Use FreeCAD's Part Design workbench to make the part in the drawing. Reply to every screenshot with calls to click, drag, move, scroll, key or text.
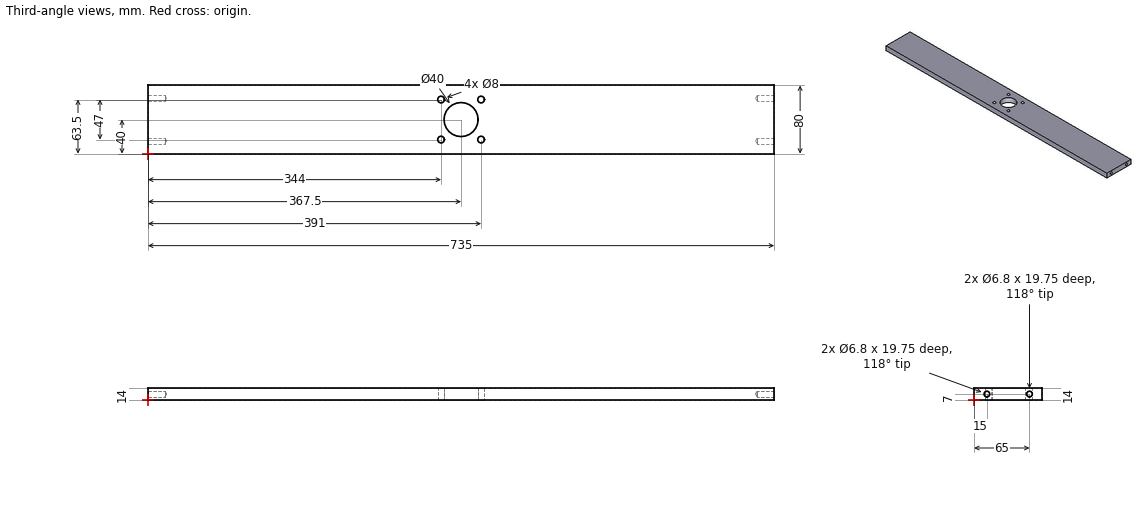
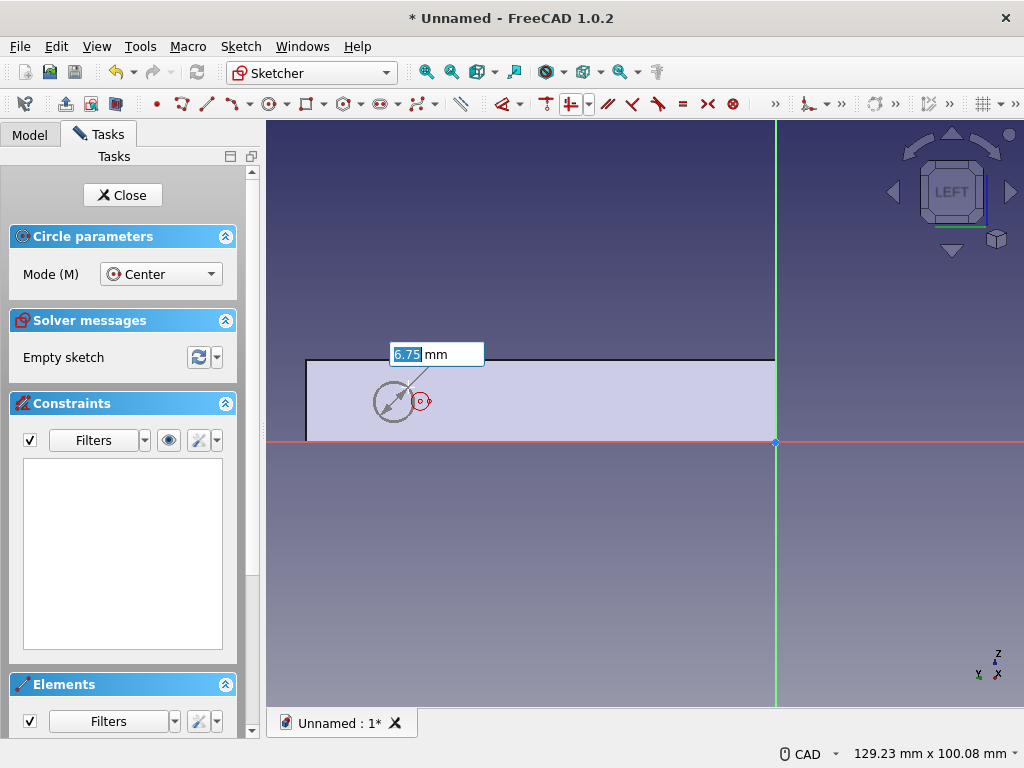
text(6.8)
key(Return)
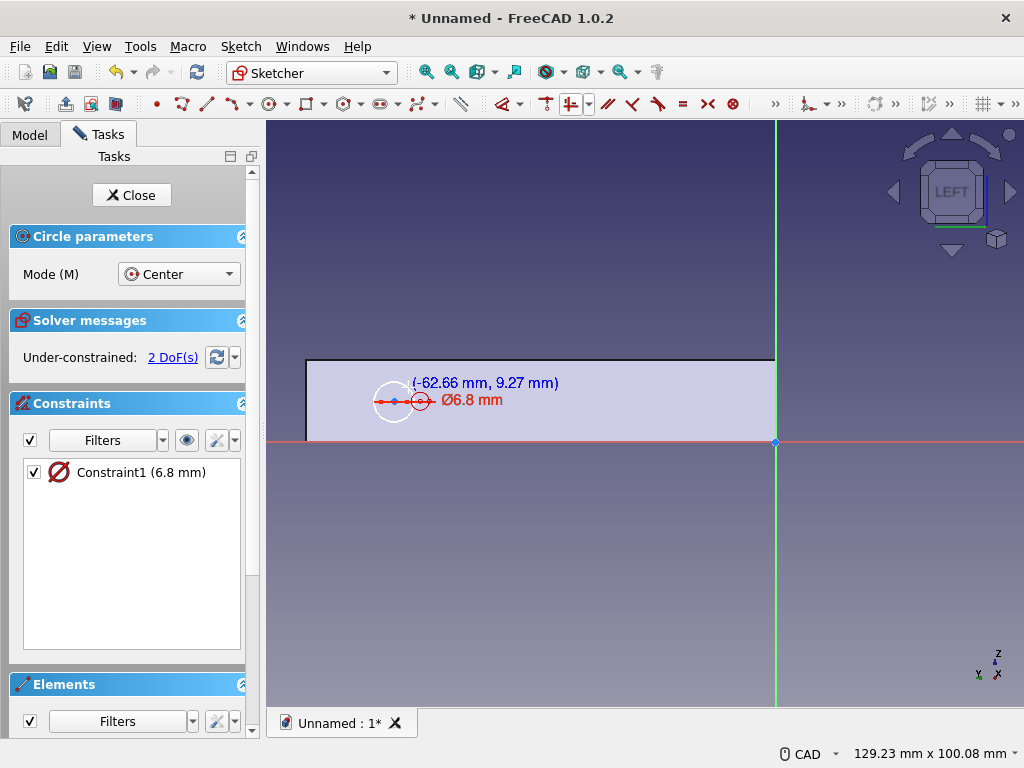
click(688, 401)
move(702, 387)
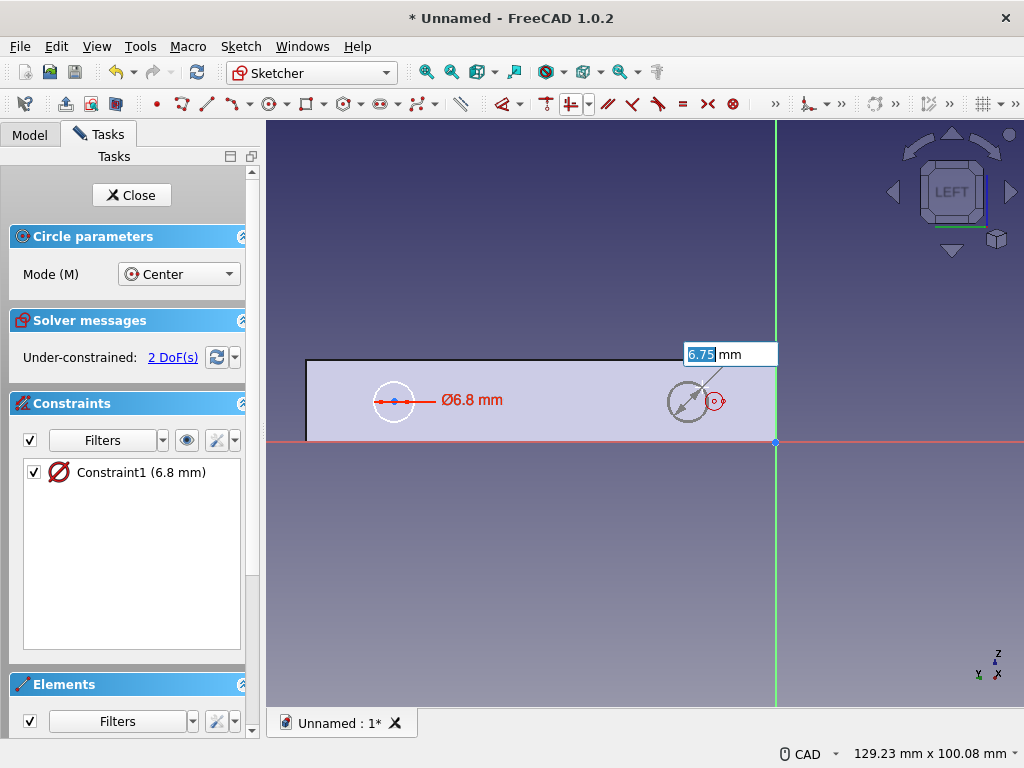
text(6.8)
key(Return)
key(Escape)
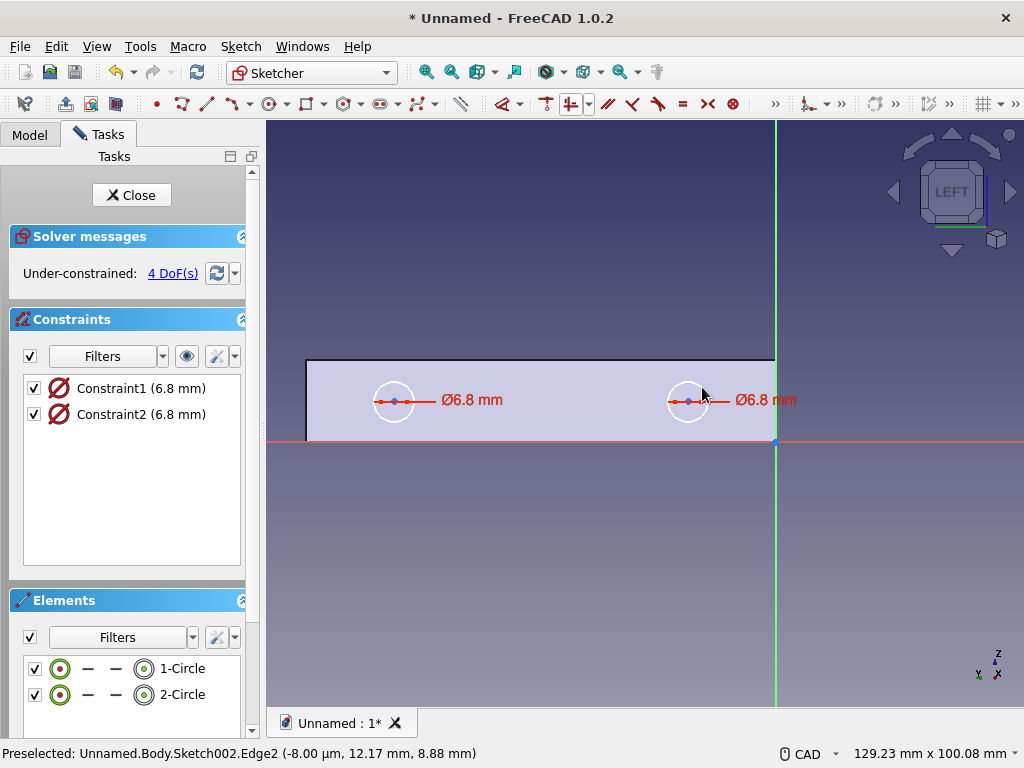
click(394, 402)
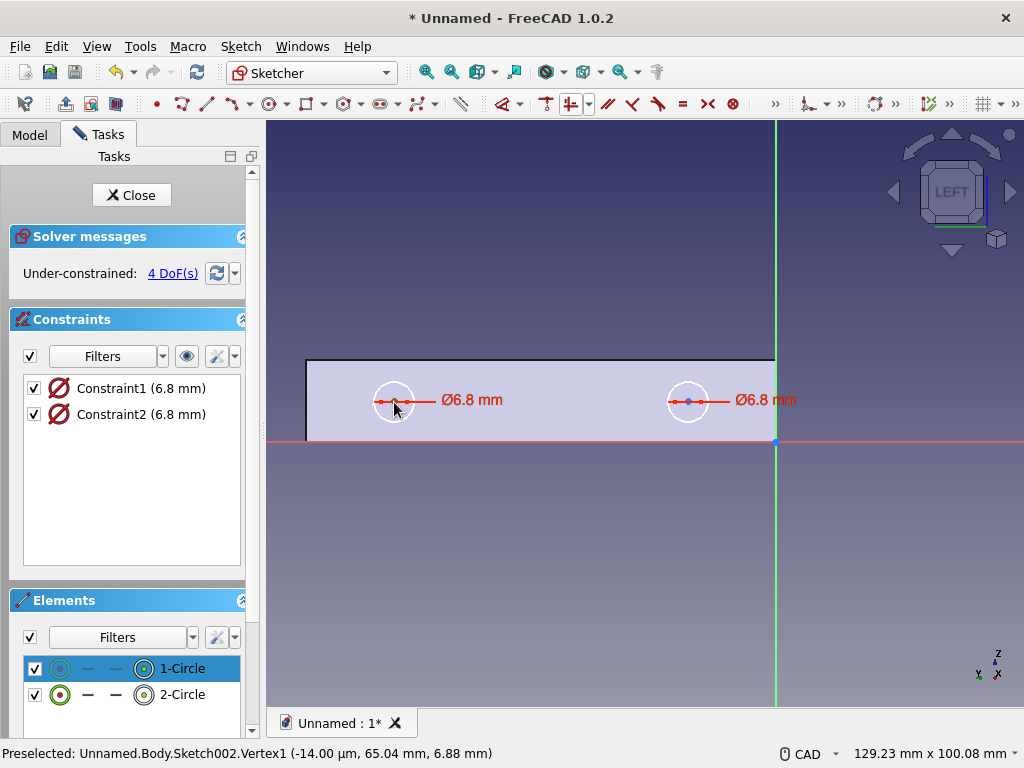
click(688, 402)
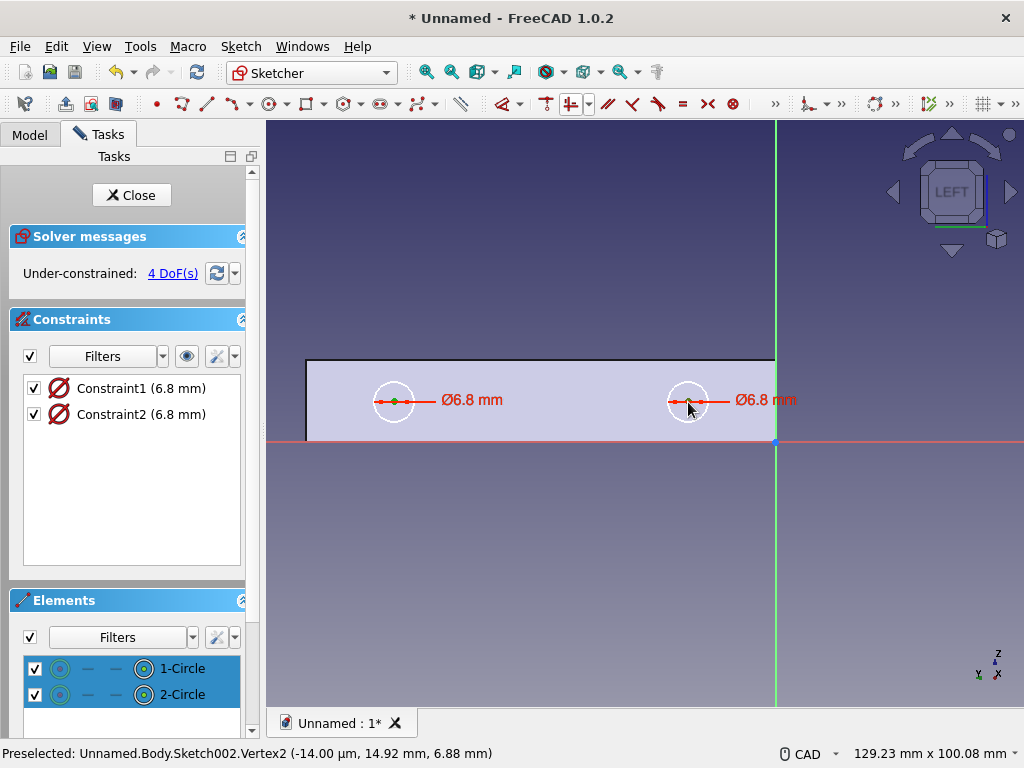
key(h)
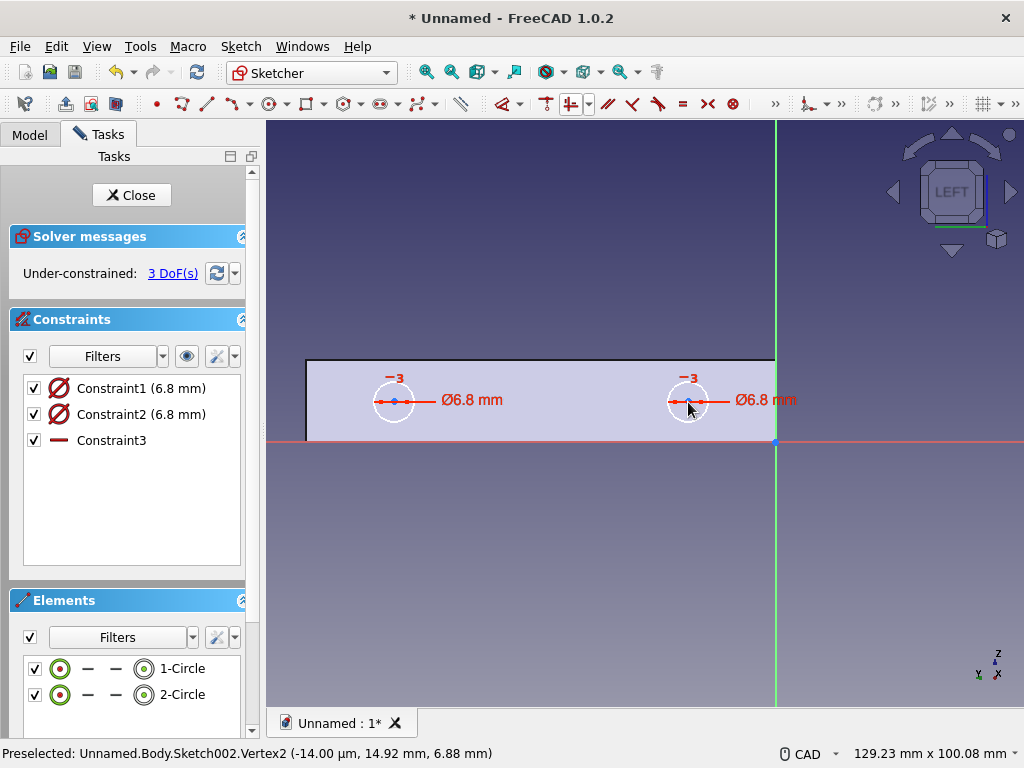
key(d)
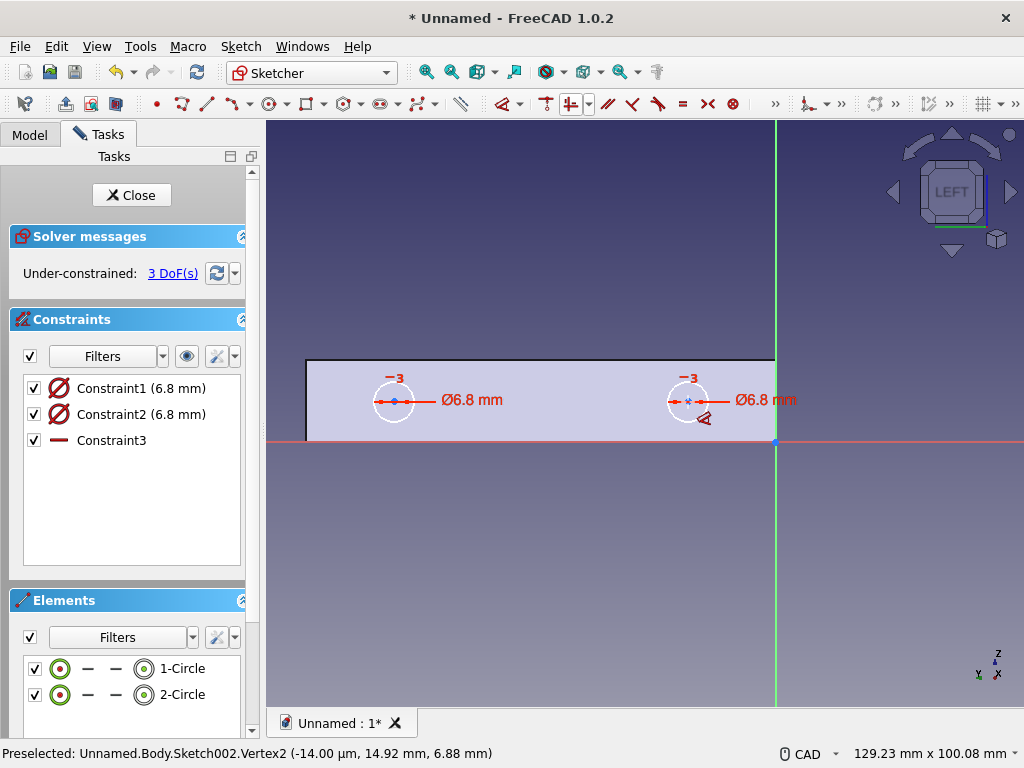
click(394, 402)
click(810, 422)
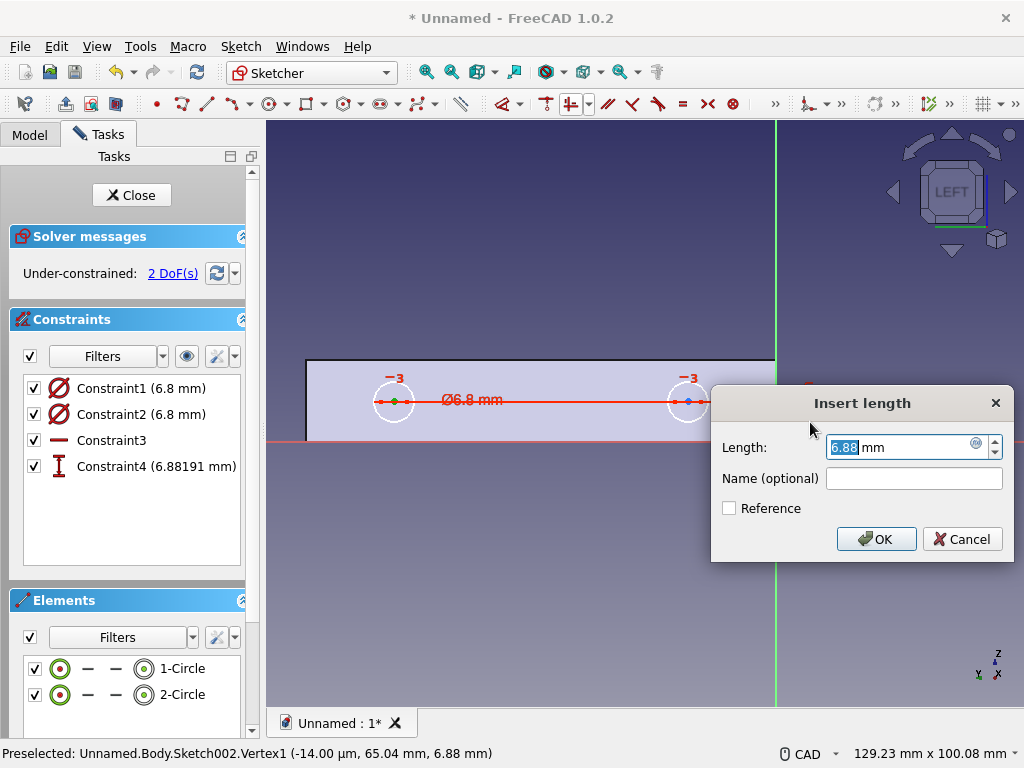
text(7)
key(Return)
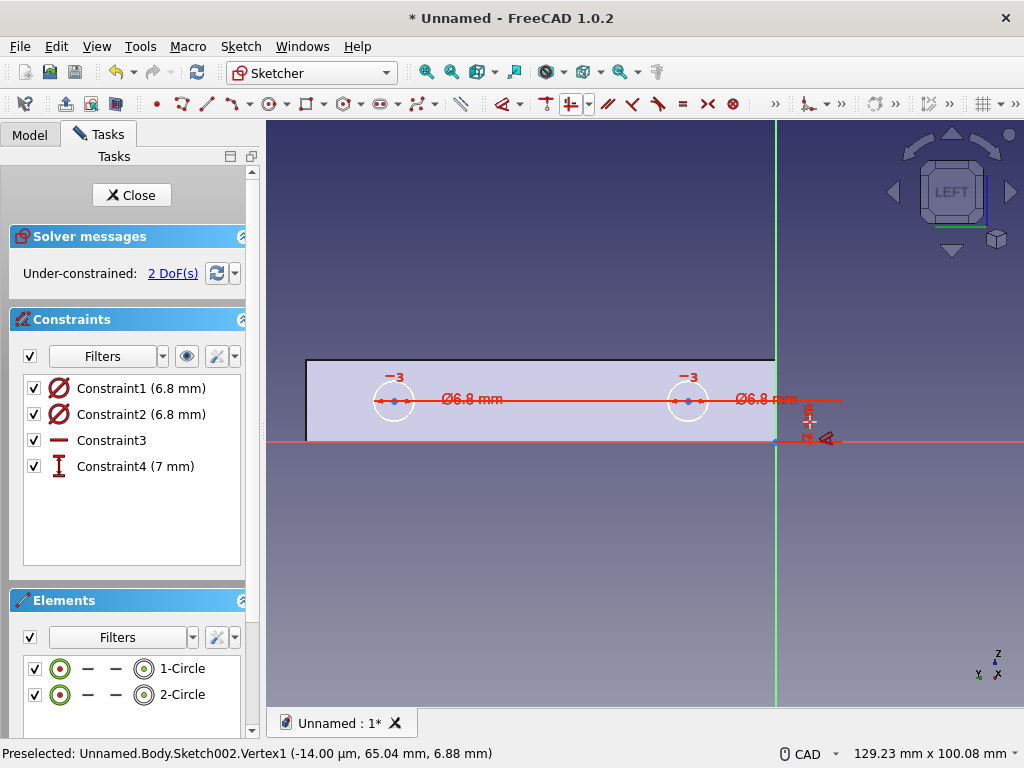
click(394, 401)
click(585, 476)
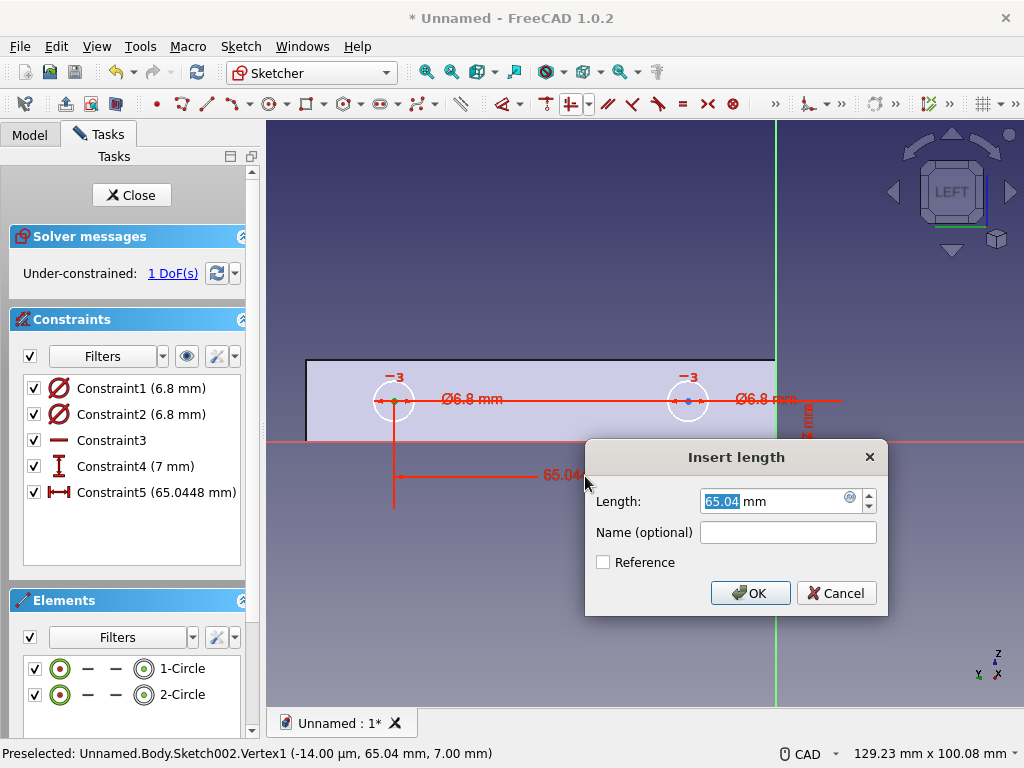
text(65)
key(Return)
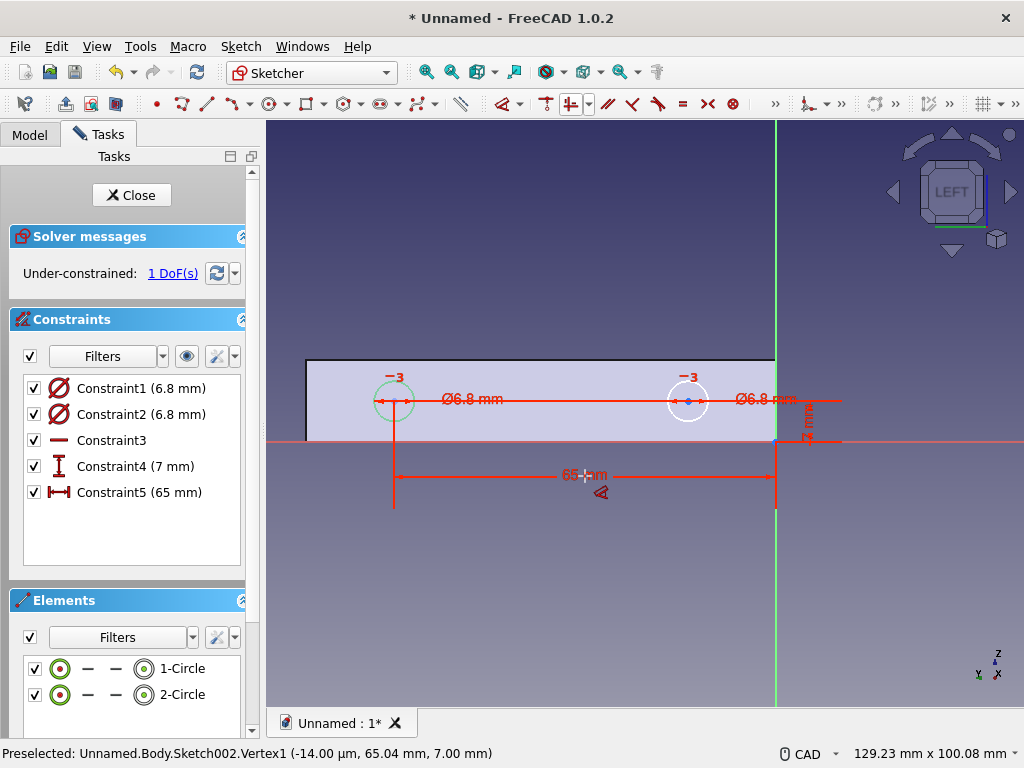
click(688, 401)
click(732, 476)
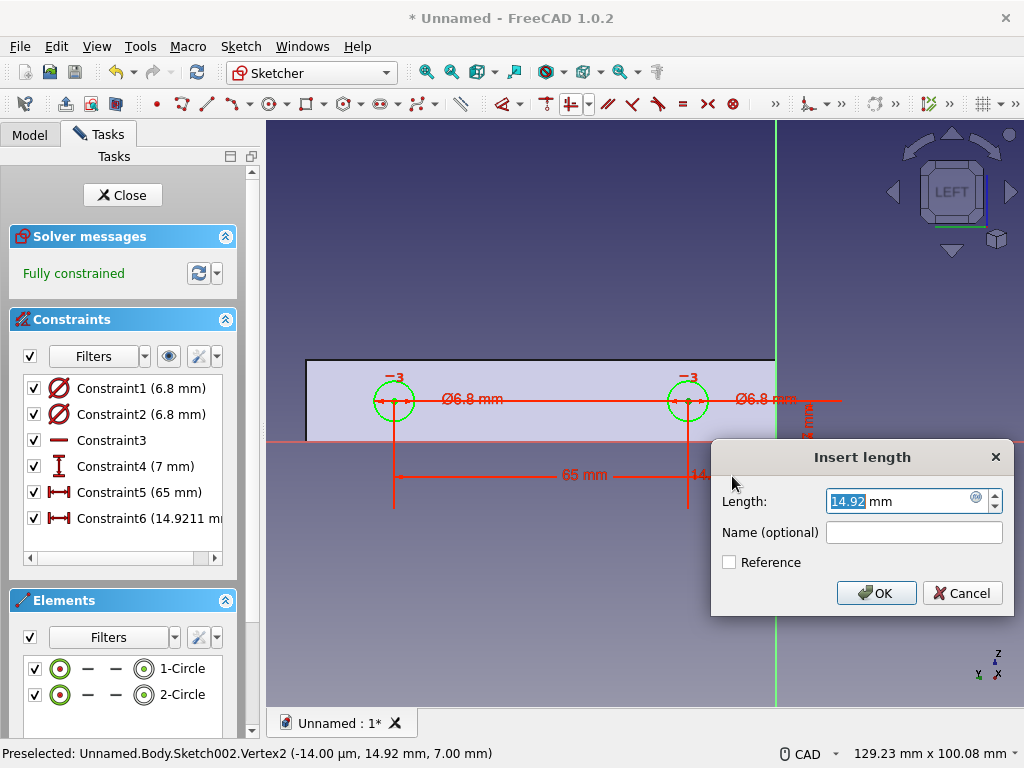
text(15)
key(Return)
key(Escape)